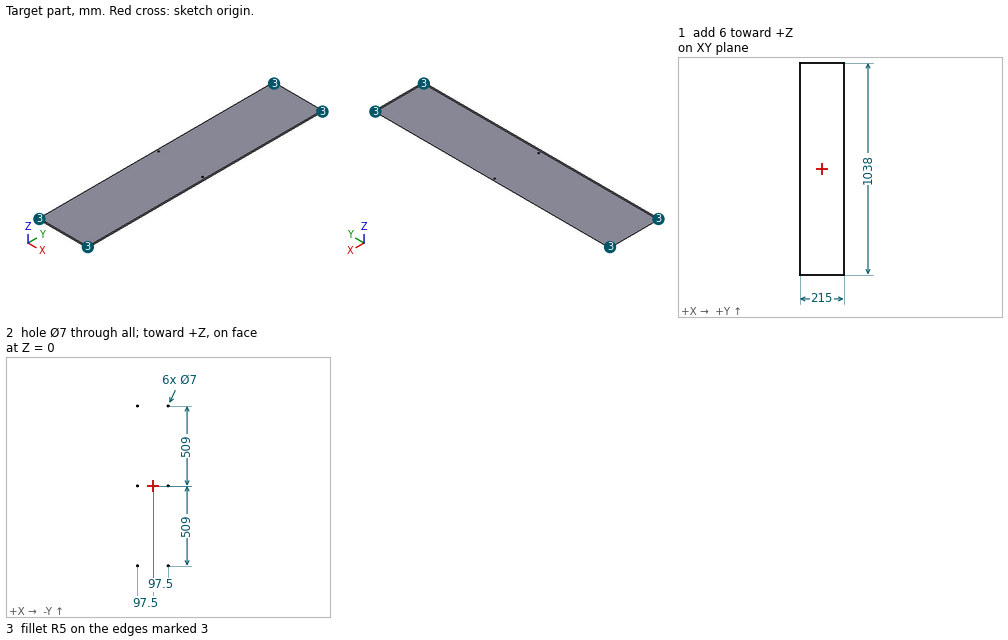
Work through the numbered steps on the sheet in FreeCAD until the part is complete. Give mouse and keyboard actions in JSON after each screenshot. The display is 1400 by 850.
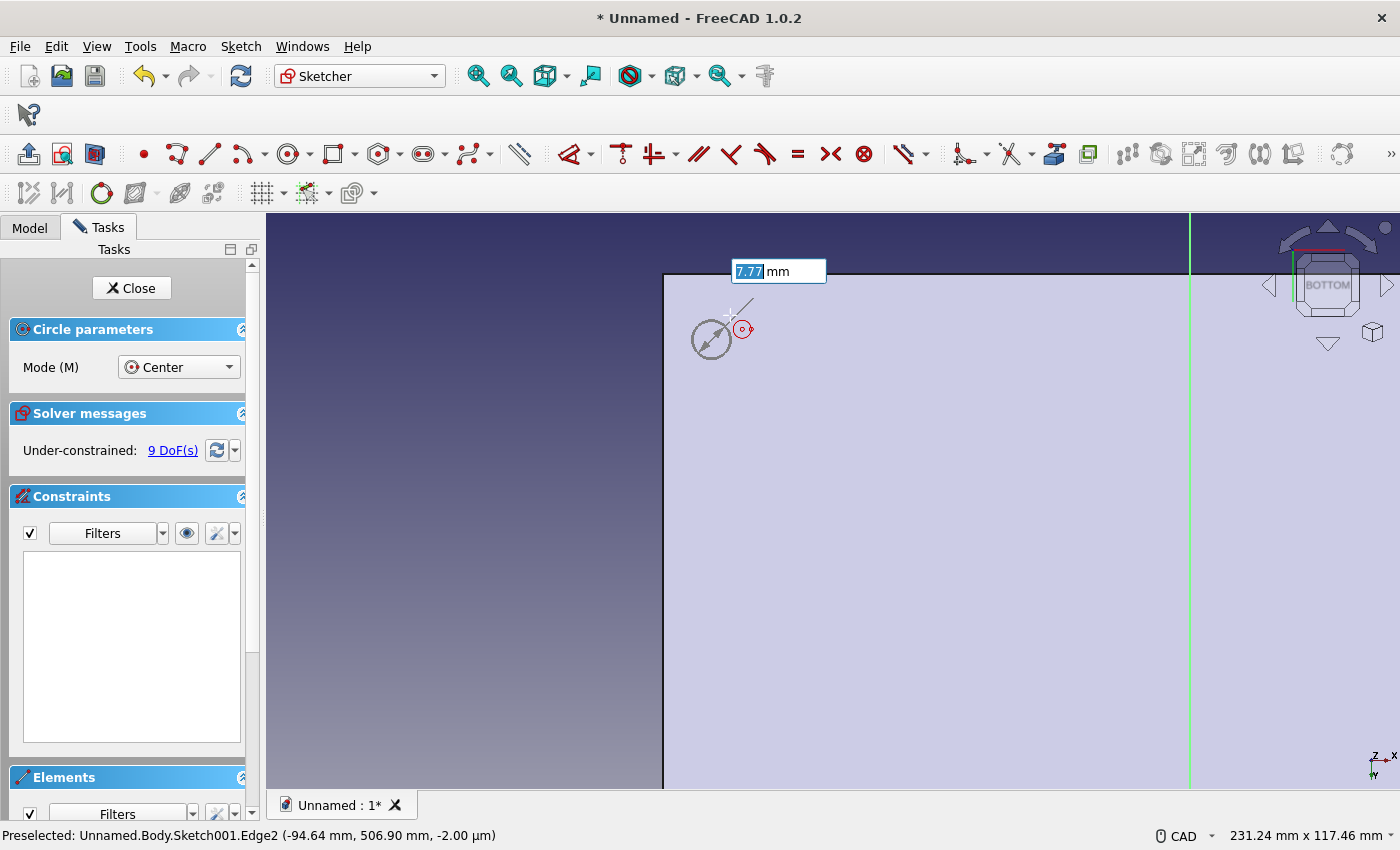
{"action": "left_click", "coordinate": [724, 311]}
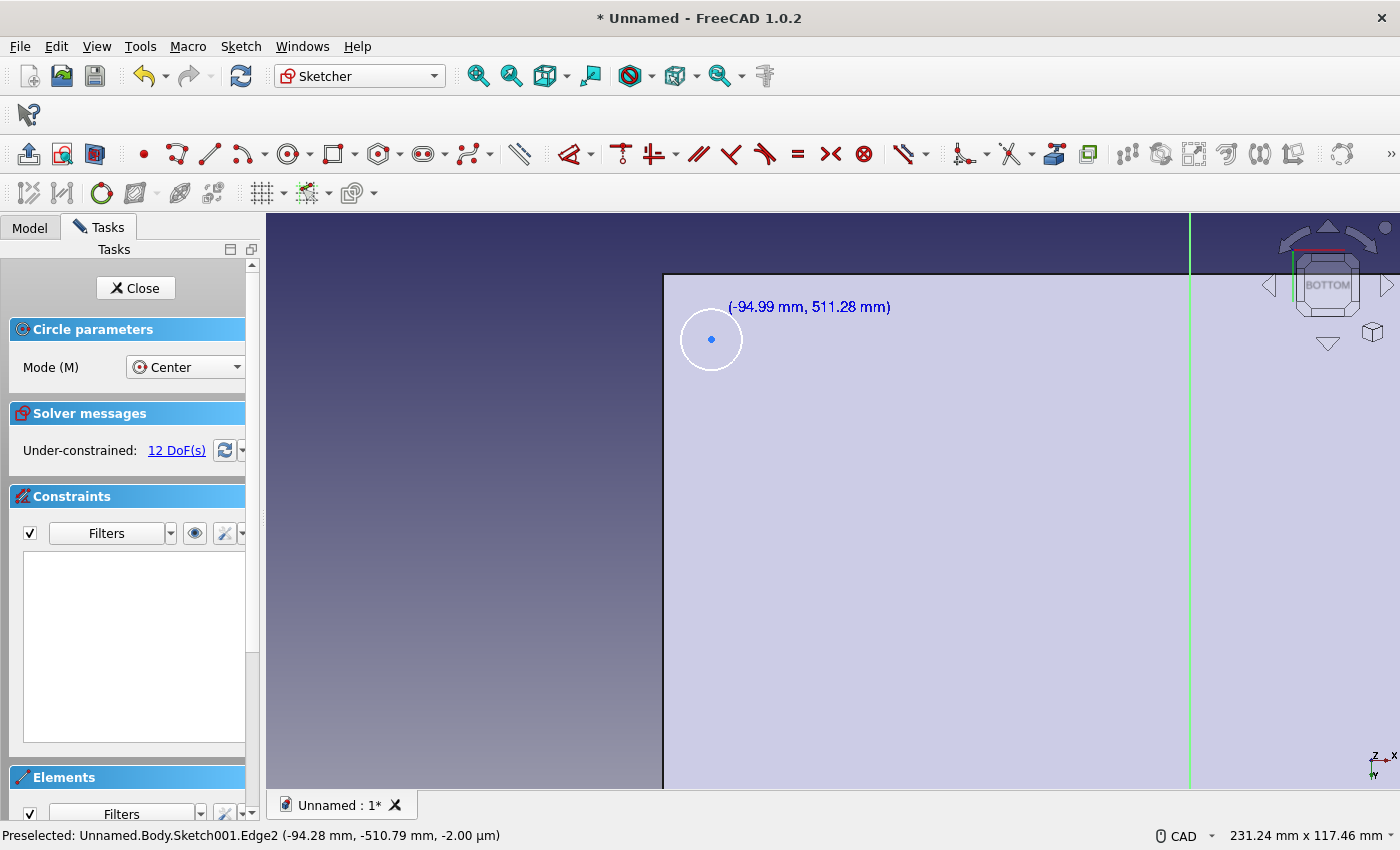
{"action": "scroll", "coordinate": [730, 315], "scroll_direction": "down", "scroll_amount": 13}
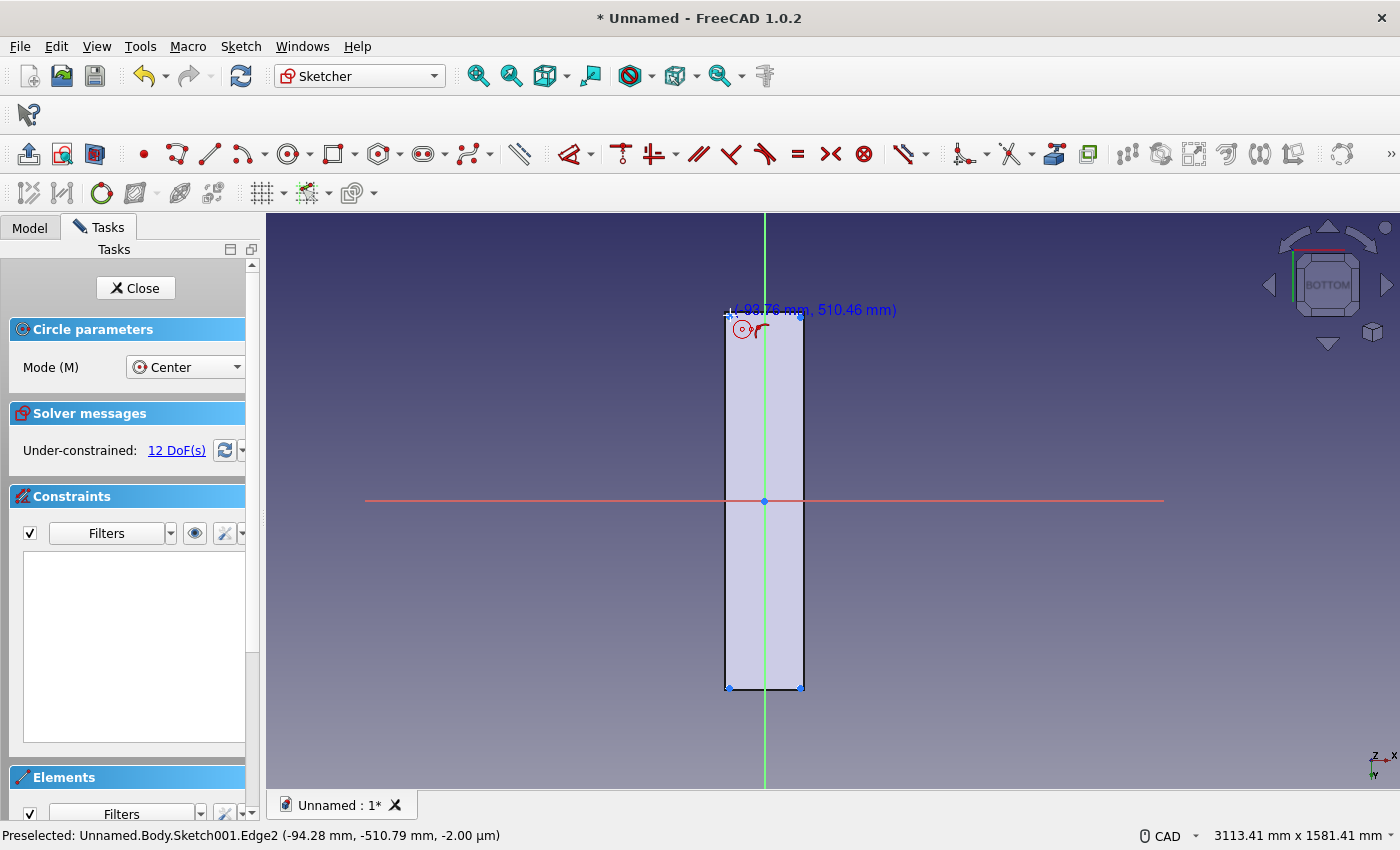
{"action": "scroll", "coordinate": [800, 501], "scroll_direction": "up", "scroll_amount": 15}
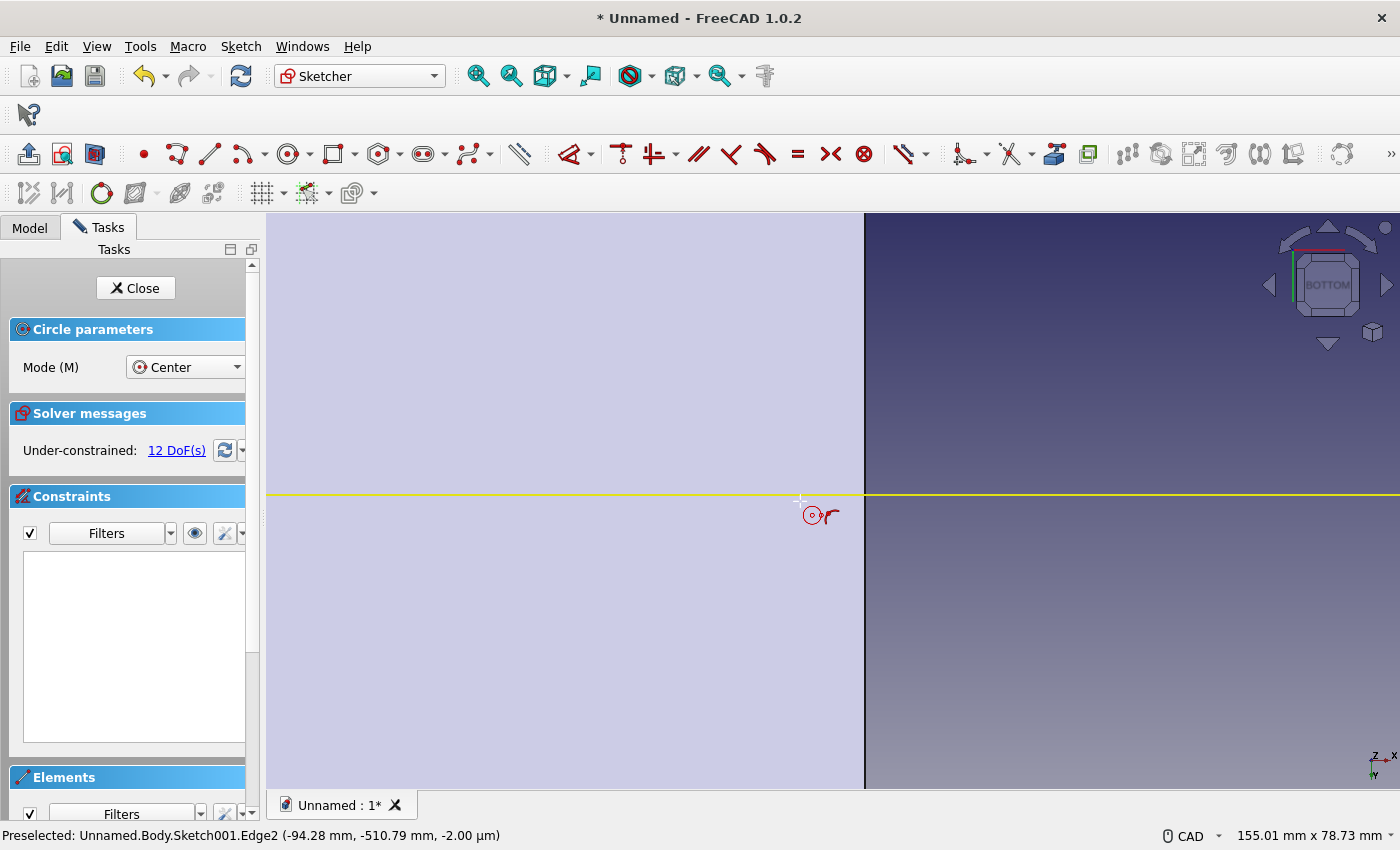
{"action": "scroll", "coordinate": [800, 501], "scroll_direction": "down", "scroll_amount": 15}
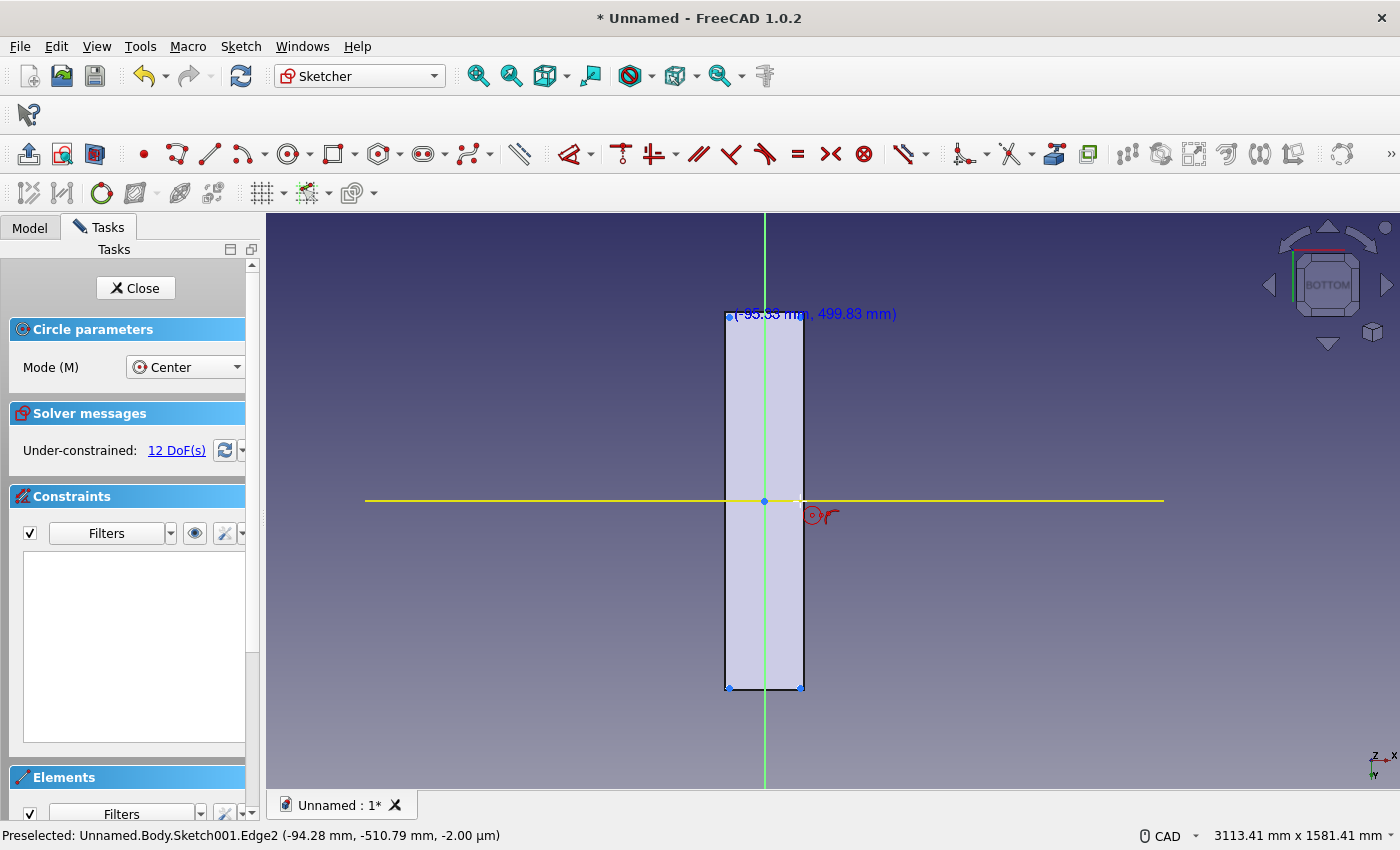
{"action": "left_click", "coordinate": [800, 501]}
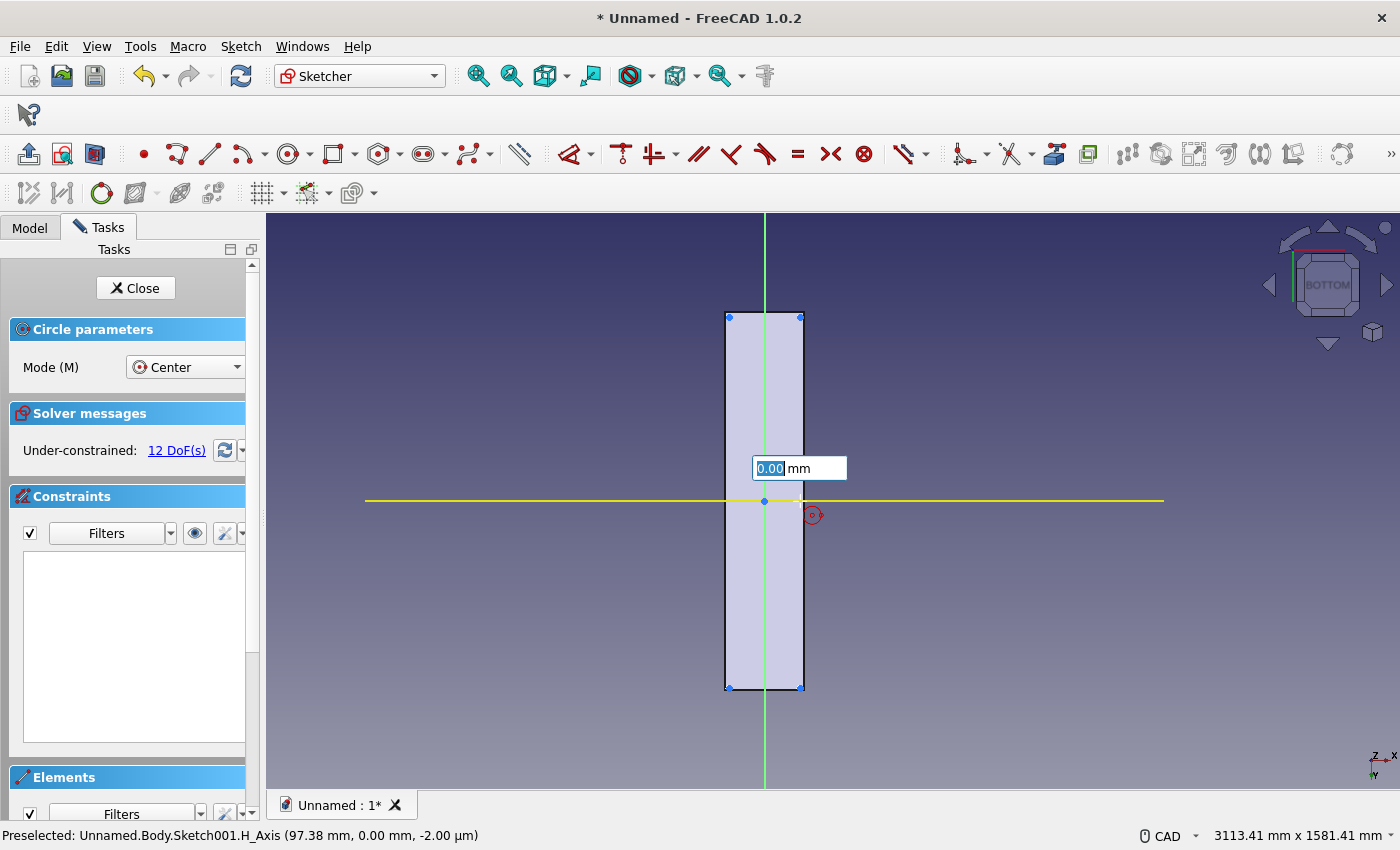
{"action": "scroll", "coordinate": [800, 500], "scroll_direction": "up", "scroll_amount": 13}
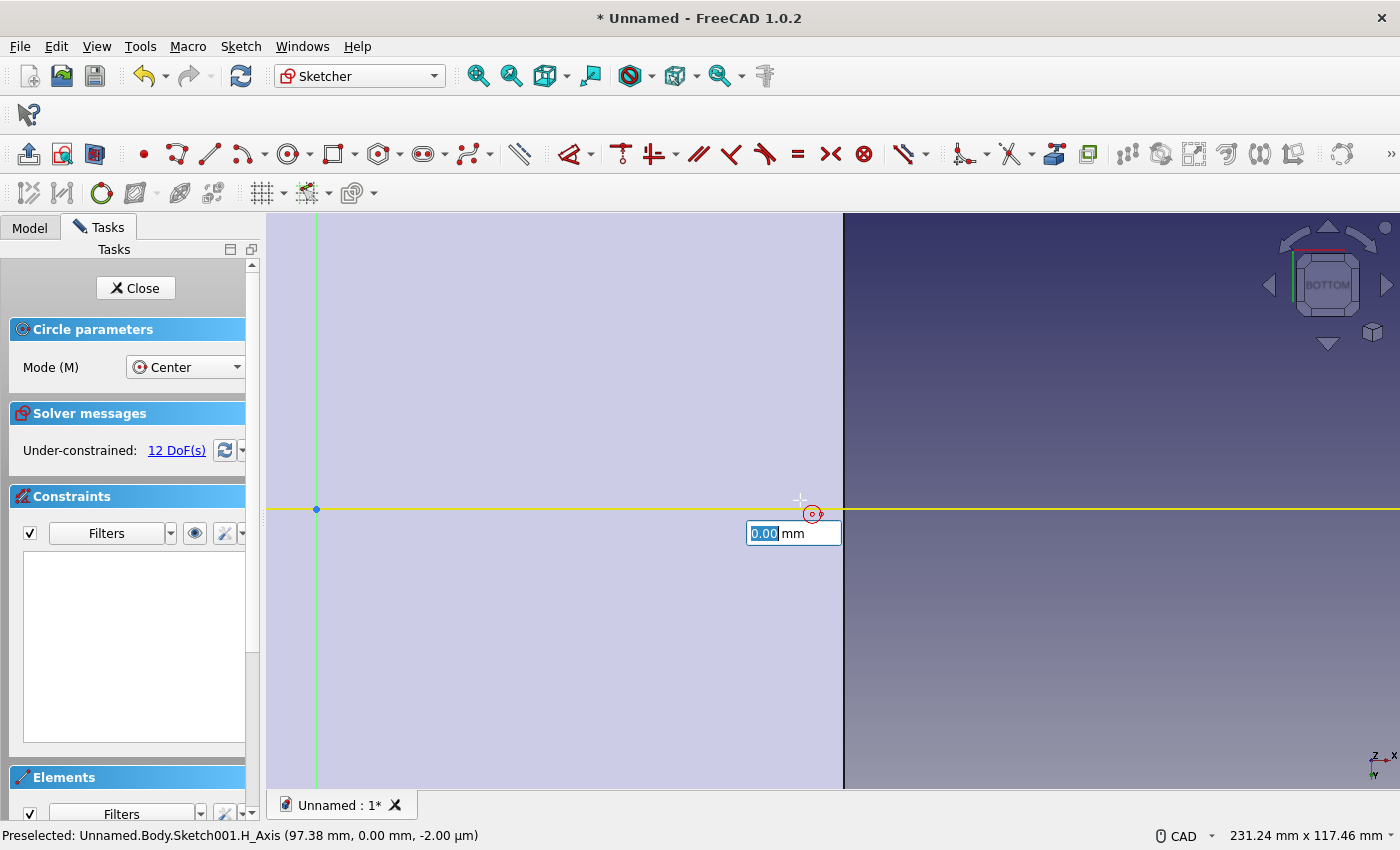
{"action": "left_click", "coordinate": [801, 493]}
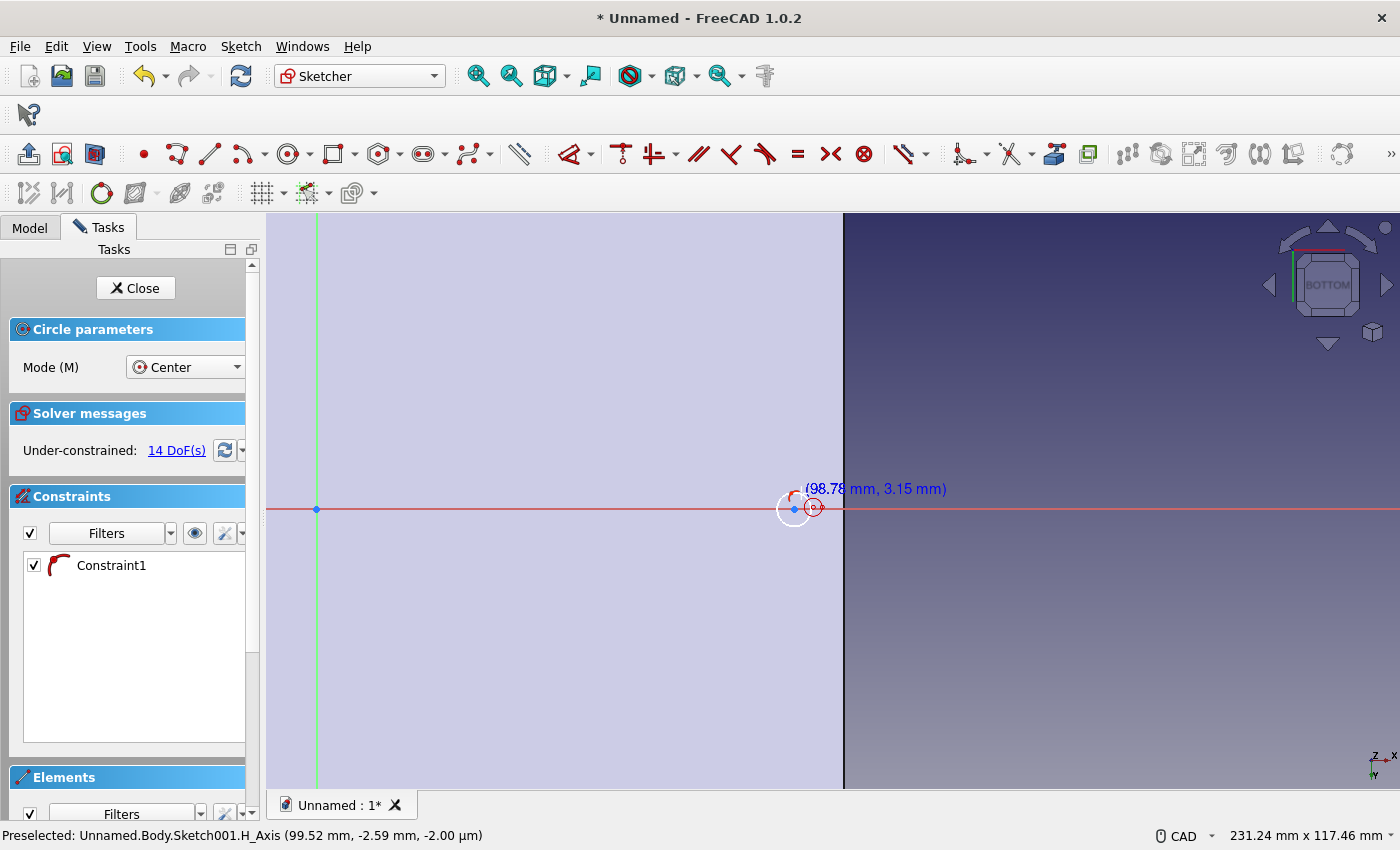
{"action": "scroll", "coordinate": [800, 500], "scroll_direction": "down", "scroll_amount": 13}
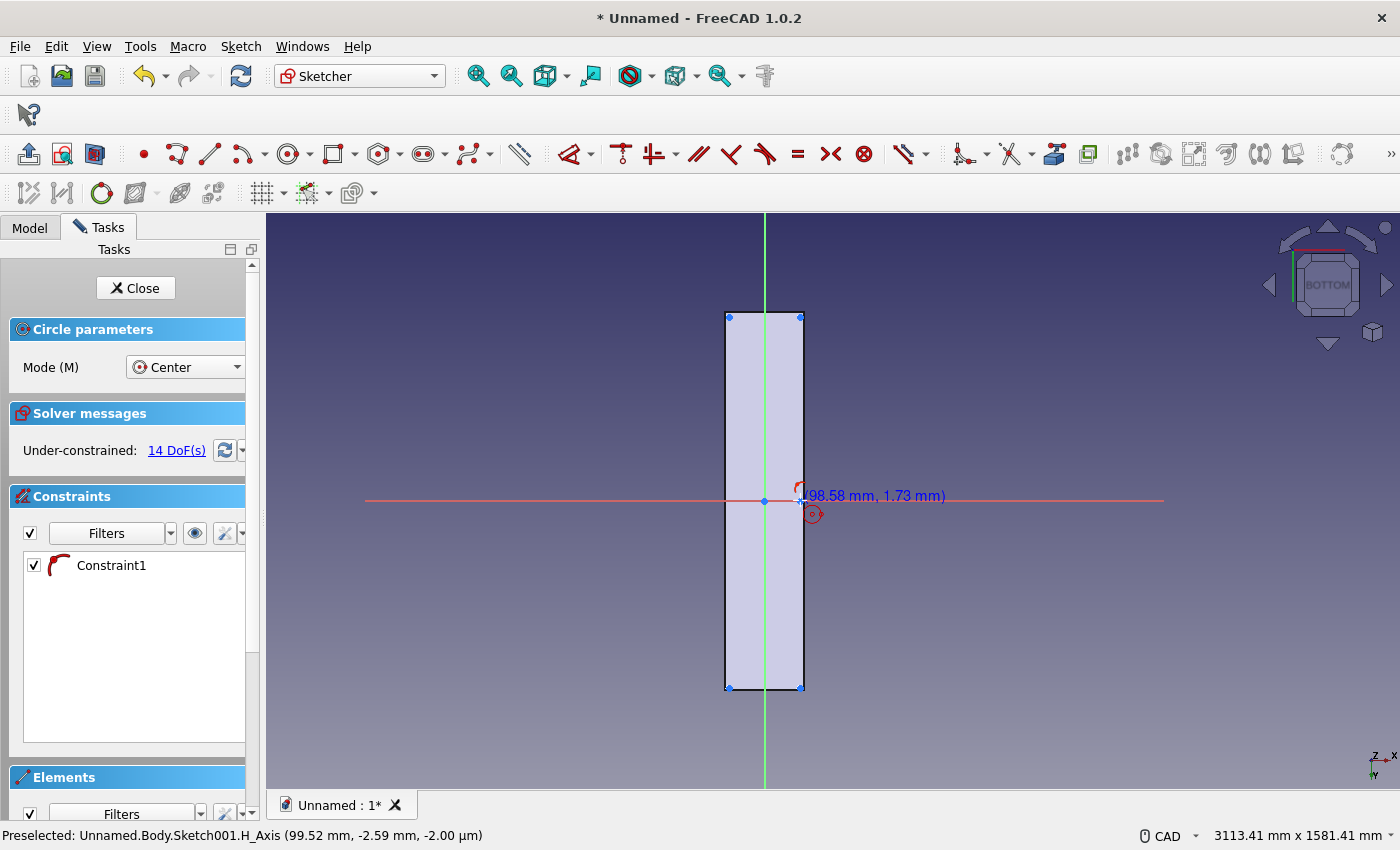
{"action": "scroll", "coordinate": [729, 501], "scroll_direction": "up", "scroll_amount": 15}